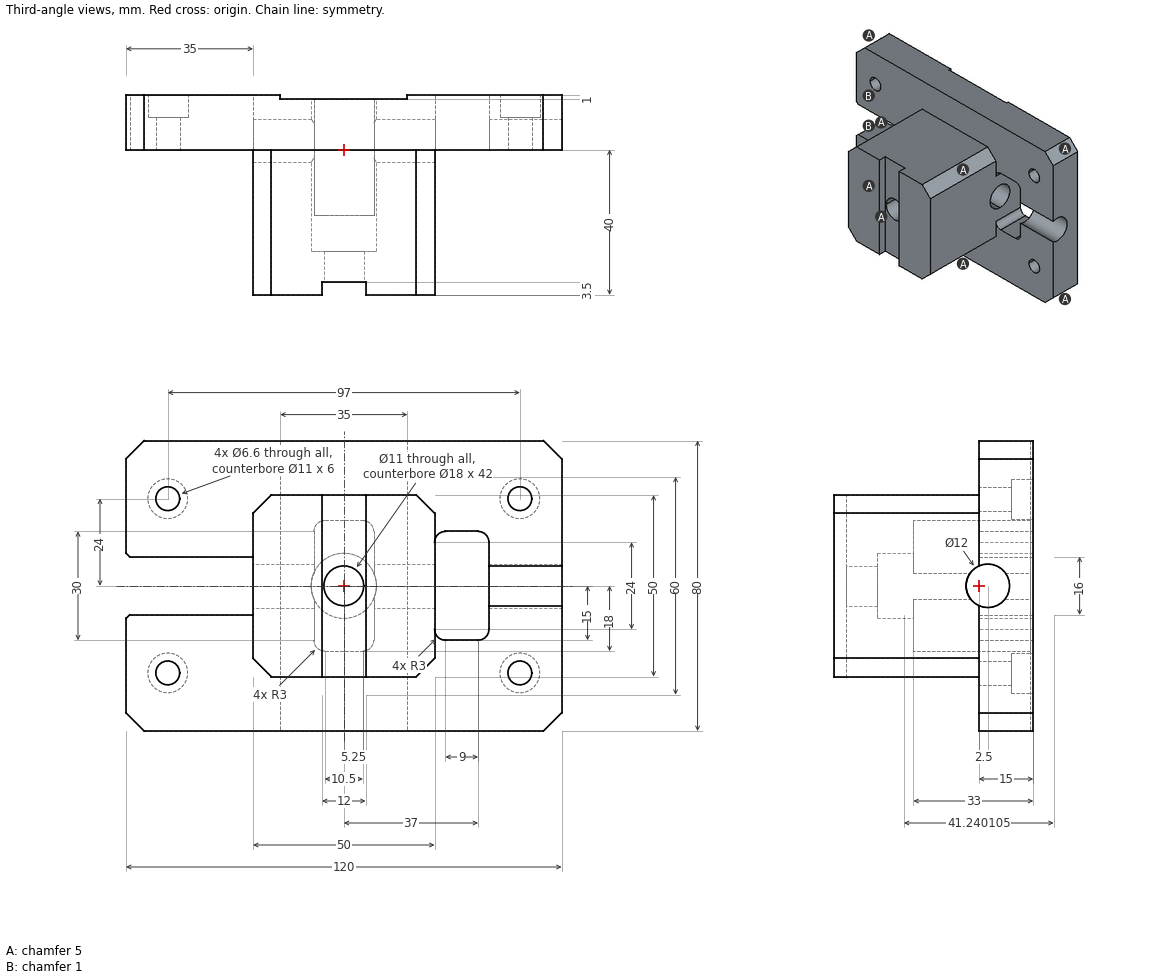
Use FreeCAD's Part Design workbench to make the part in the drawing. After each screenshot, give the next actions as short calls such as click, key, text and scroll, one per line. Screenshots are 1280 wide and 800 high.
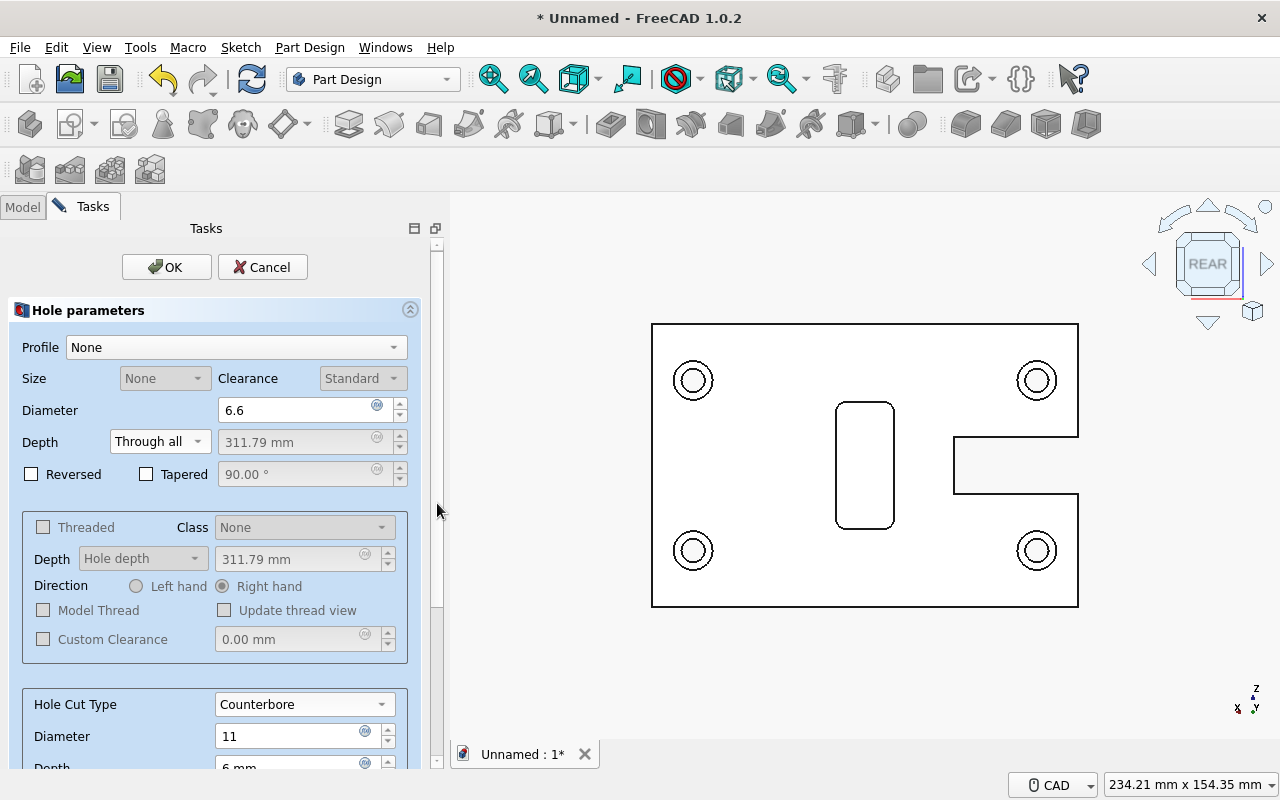
click(167, 267)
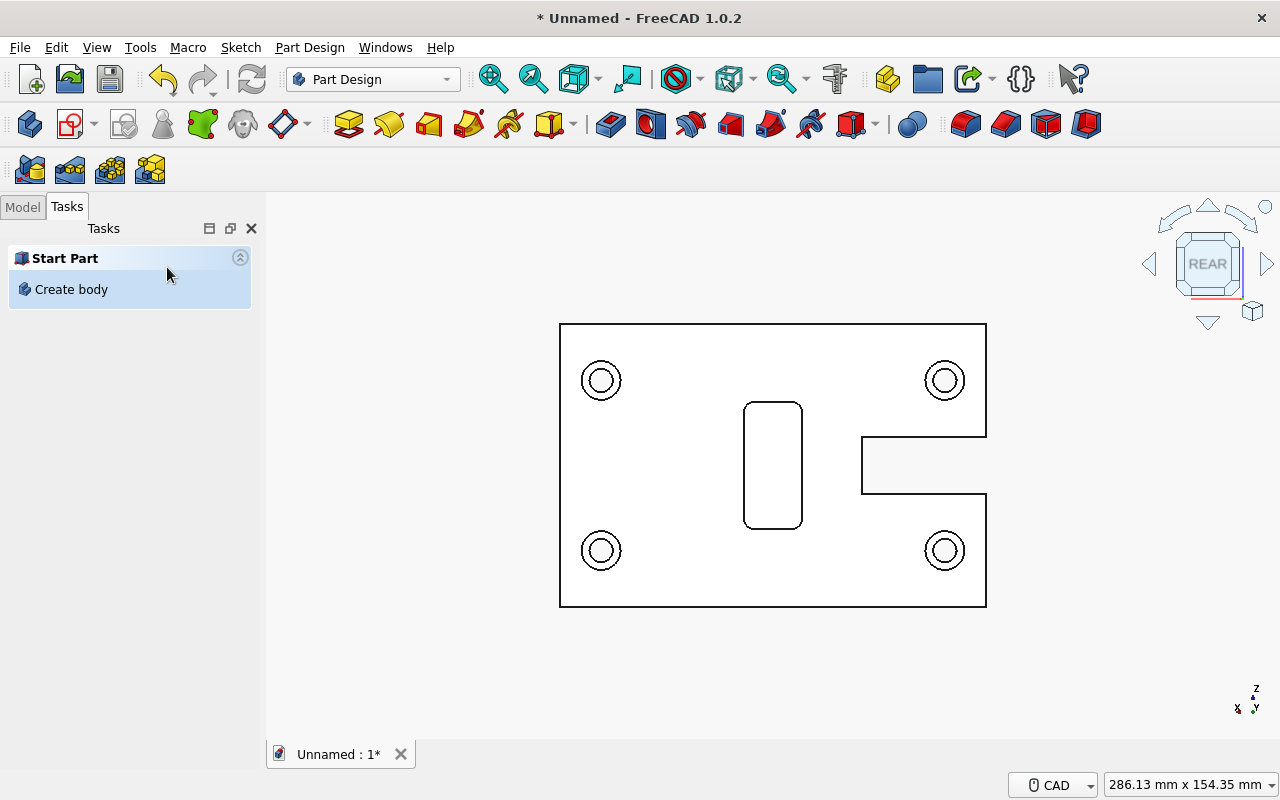
key(0)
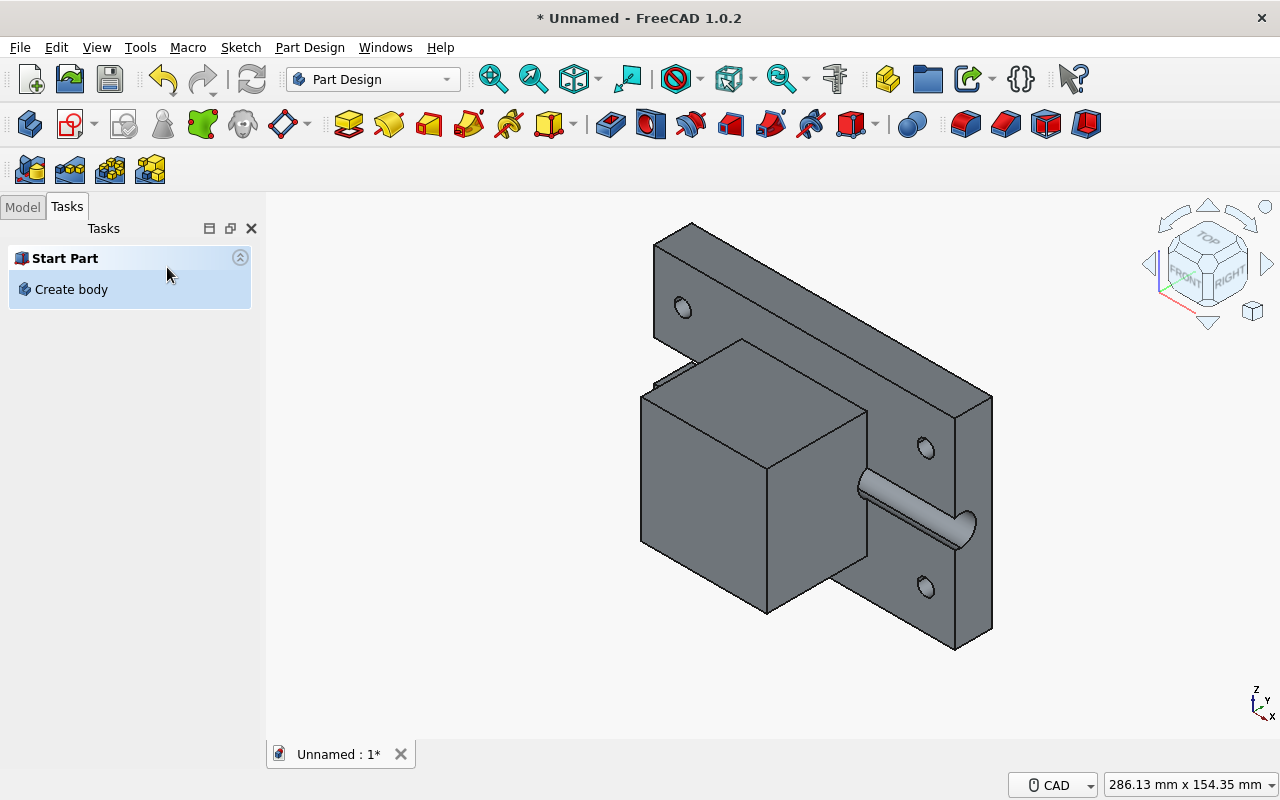
click(704, 504)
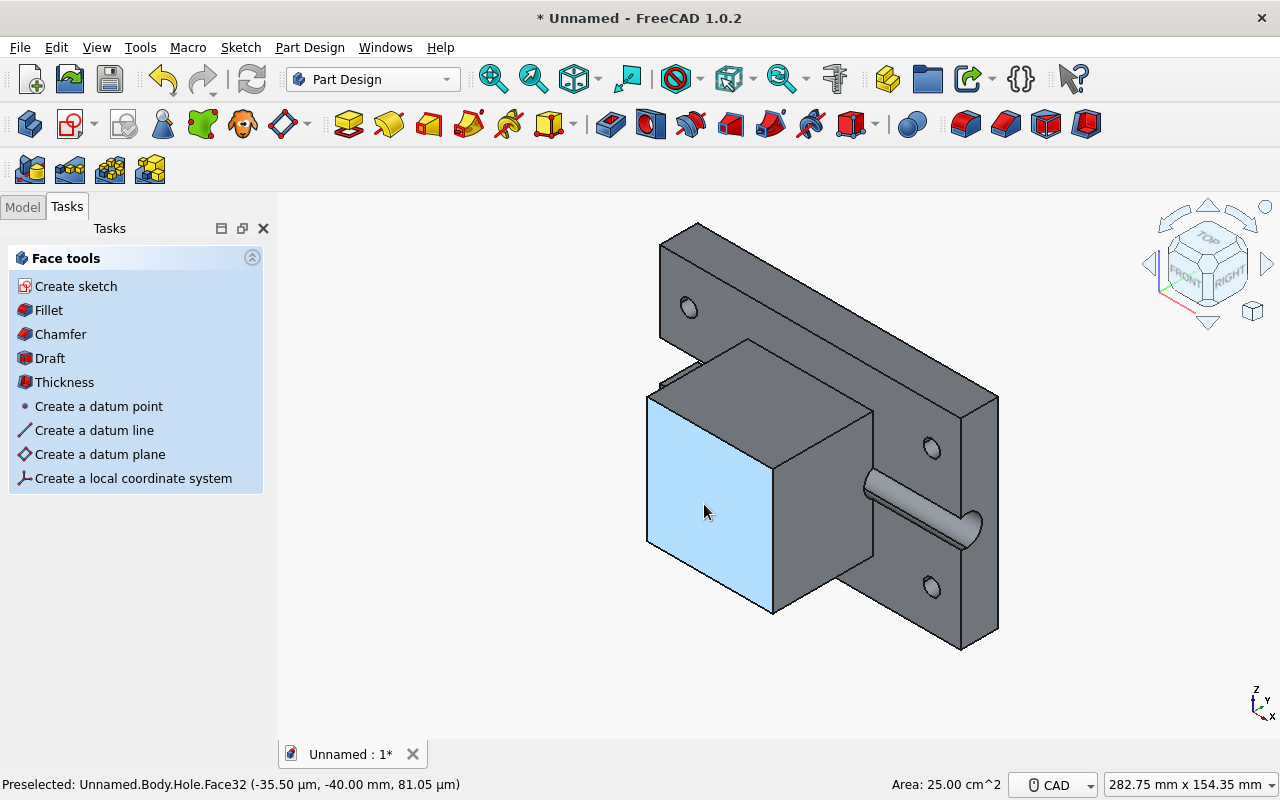
click(70, 124)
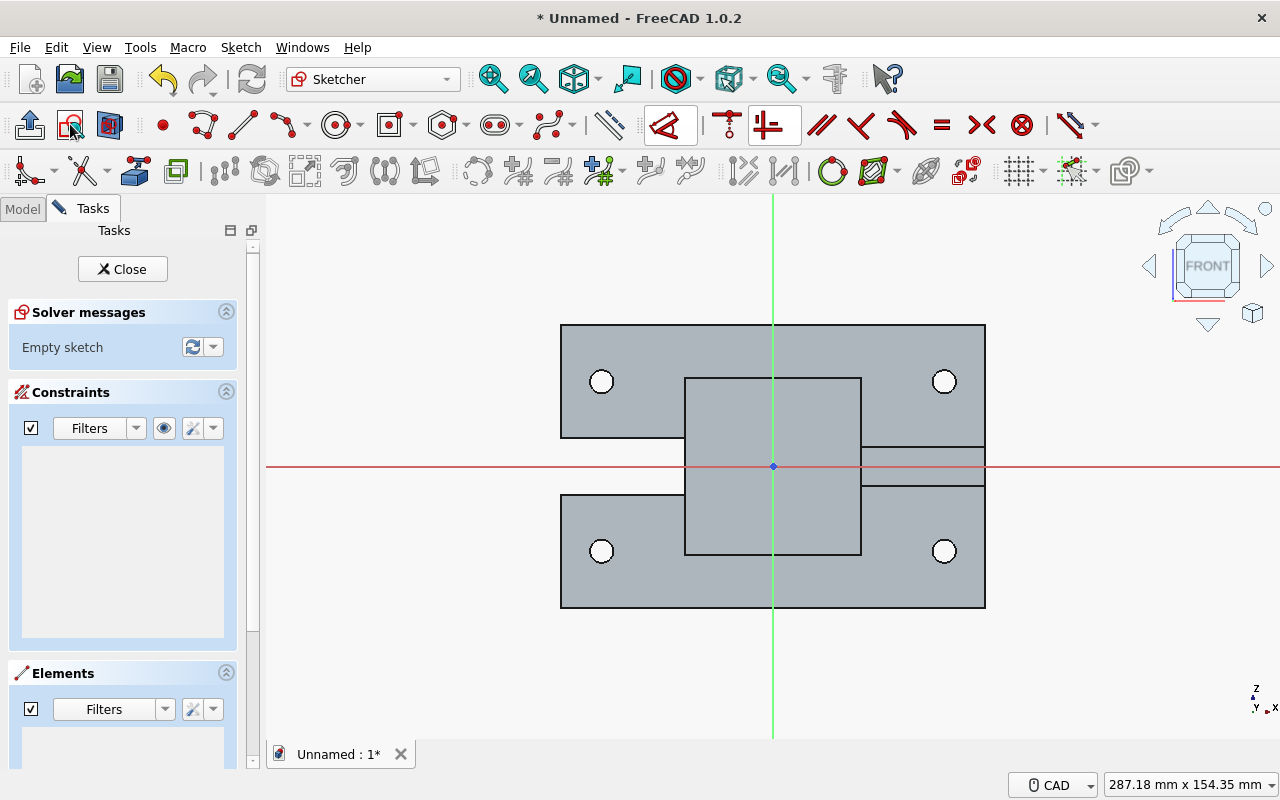
scroll(912, 467, up, 2)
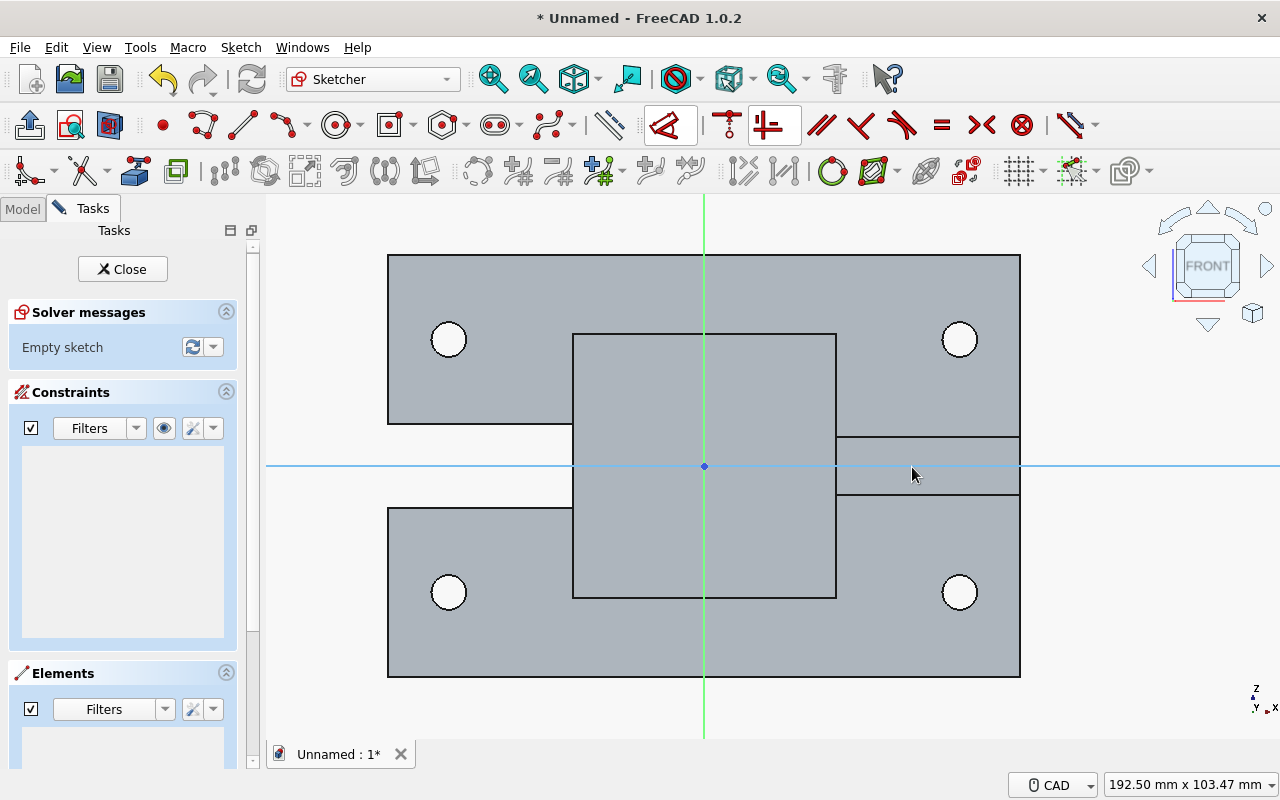
key(g)
key(v)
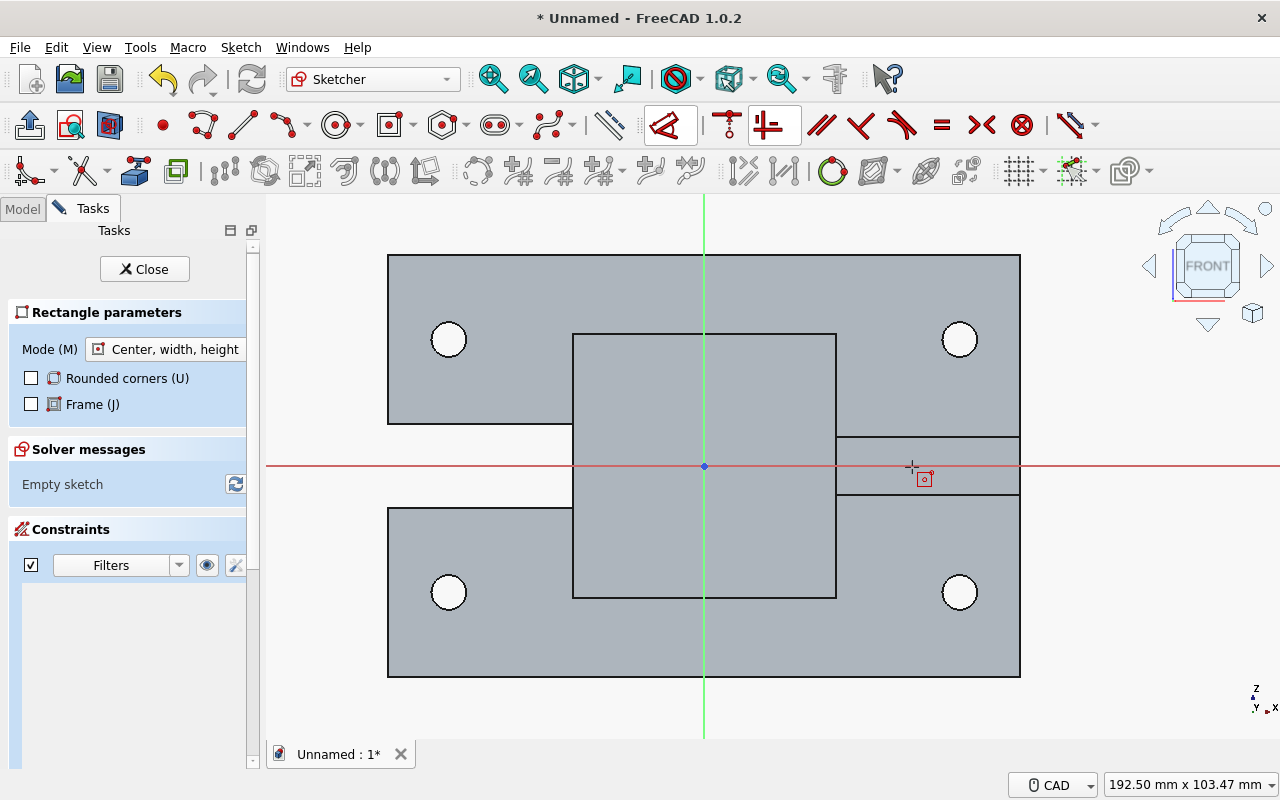
click(704, 466)
click(736, 308)
key(Escape)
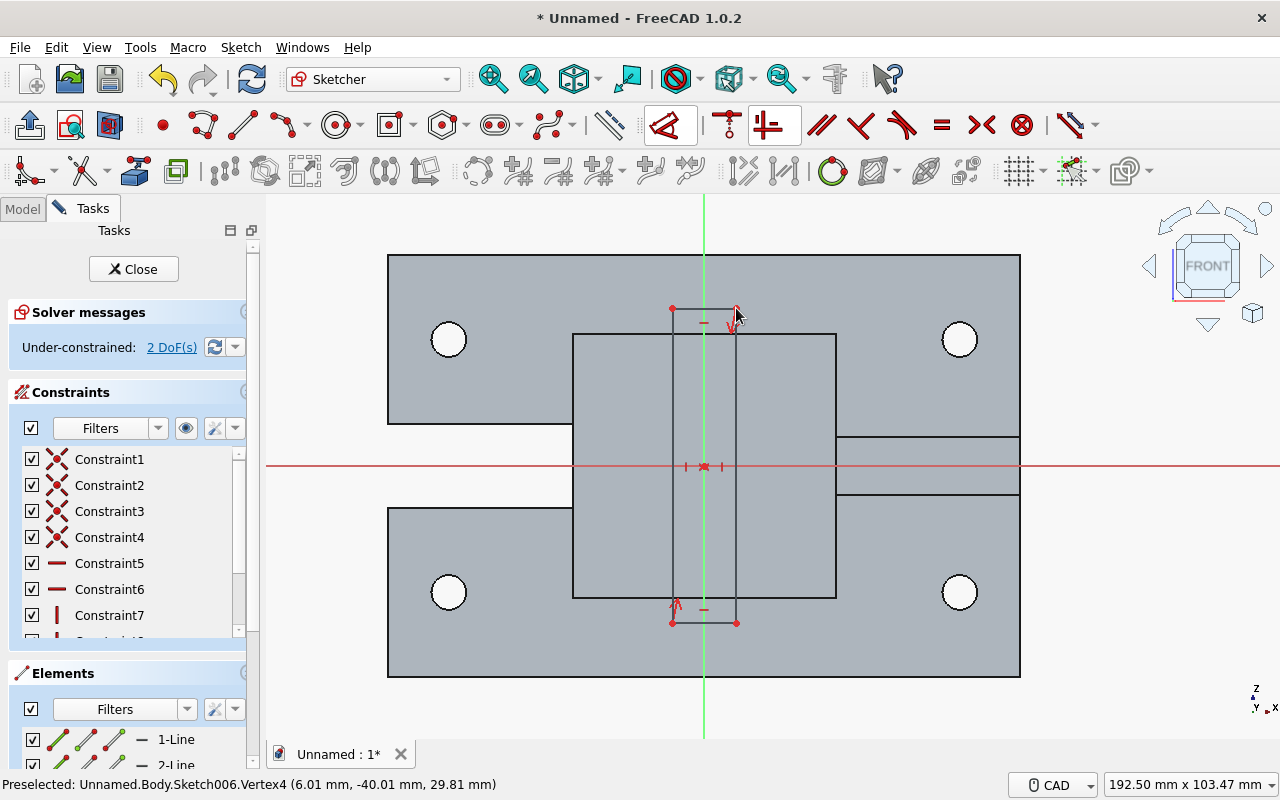
click(692, 623)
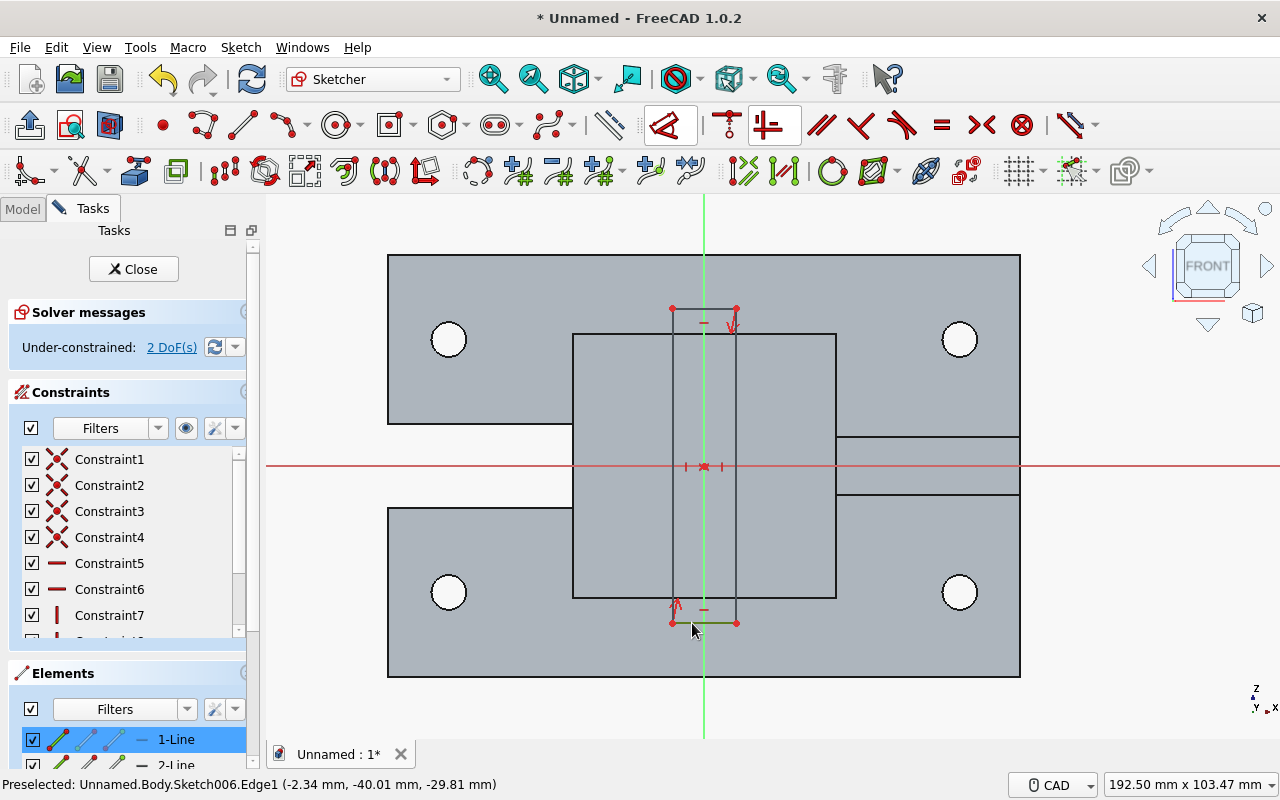
click(692, 126)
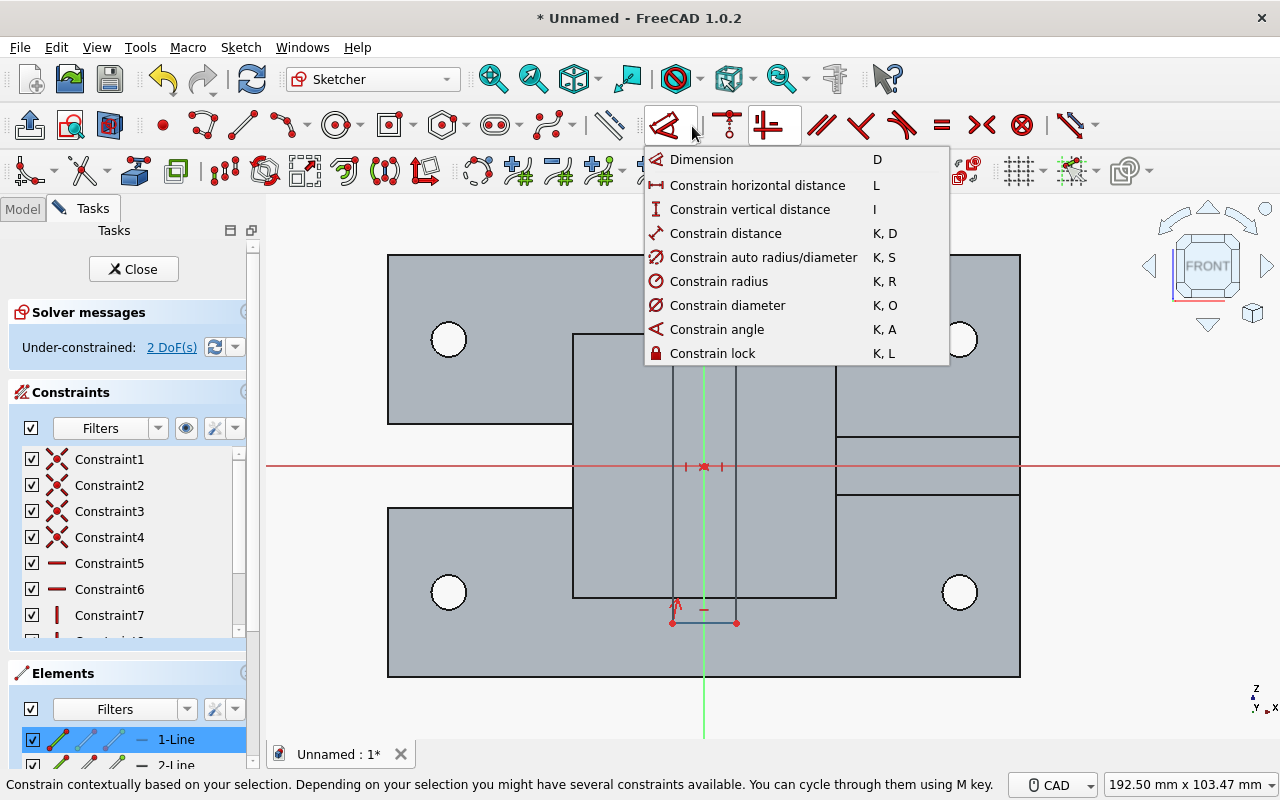
click(797, 185)